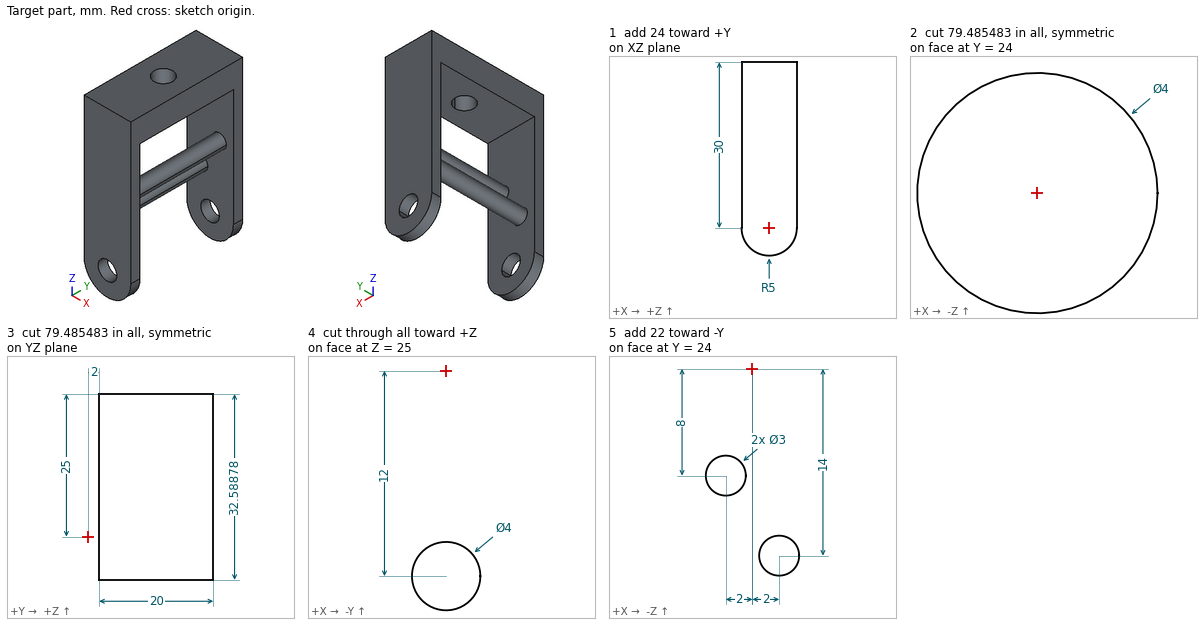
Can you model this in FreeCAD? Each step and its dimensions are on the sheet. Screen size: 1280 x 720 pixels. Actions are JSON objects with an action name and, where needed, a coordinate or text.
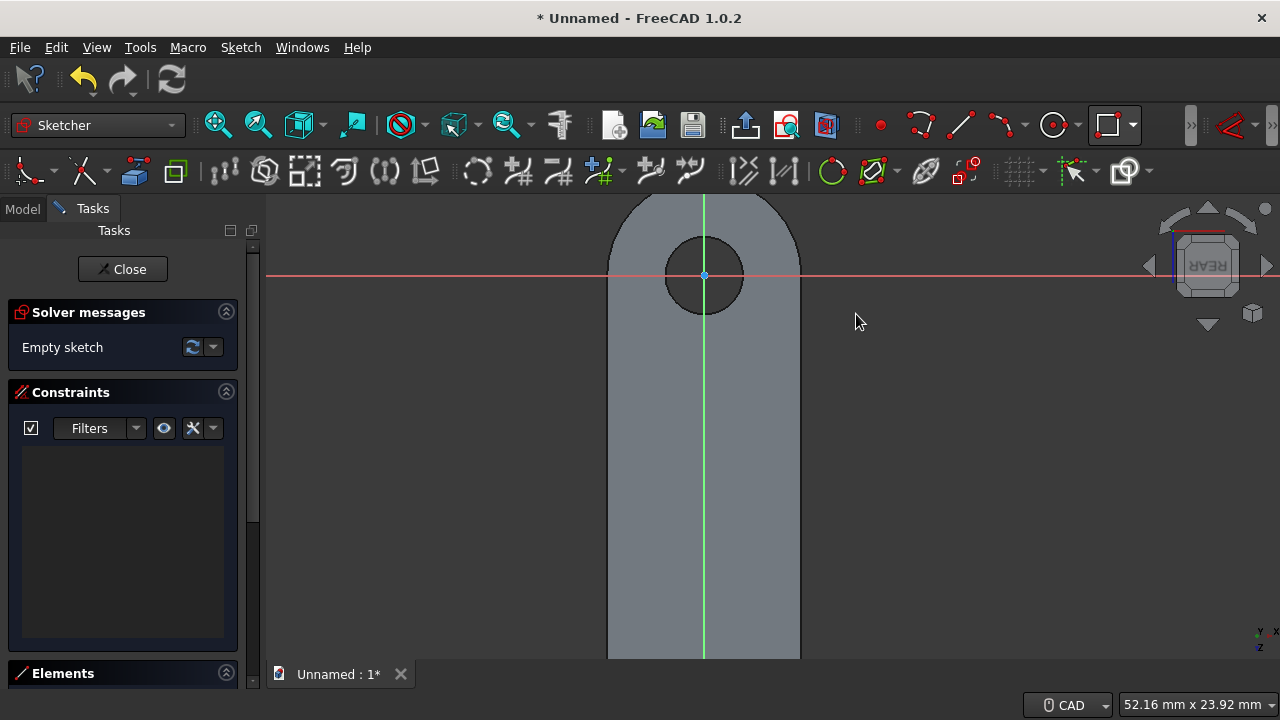
{"action": "left_click", "coordinate": [1054, 126]}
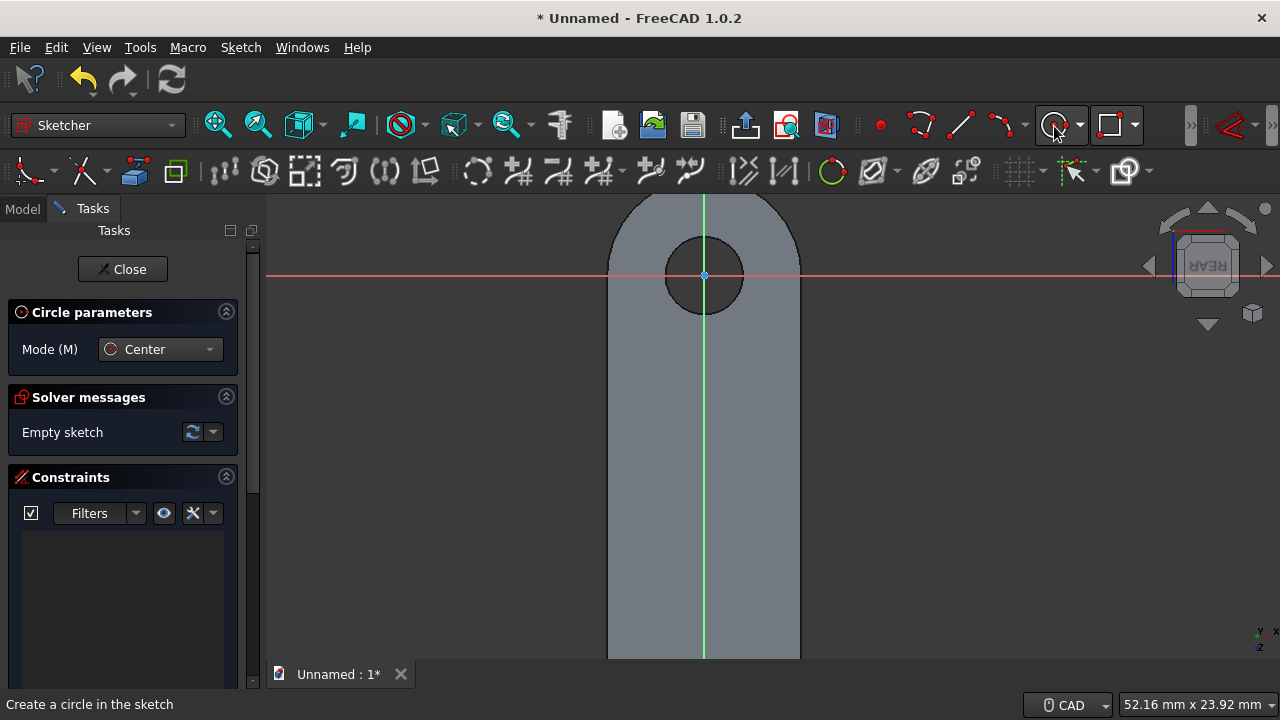
{"action": "left_click", "coordinate": [665, 431]}
{"action": "mouse_move", "coordinate": [686, 410]}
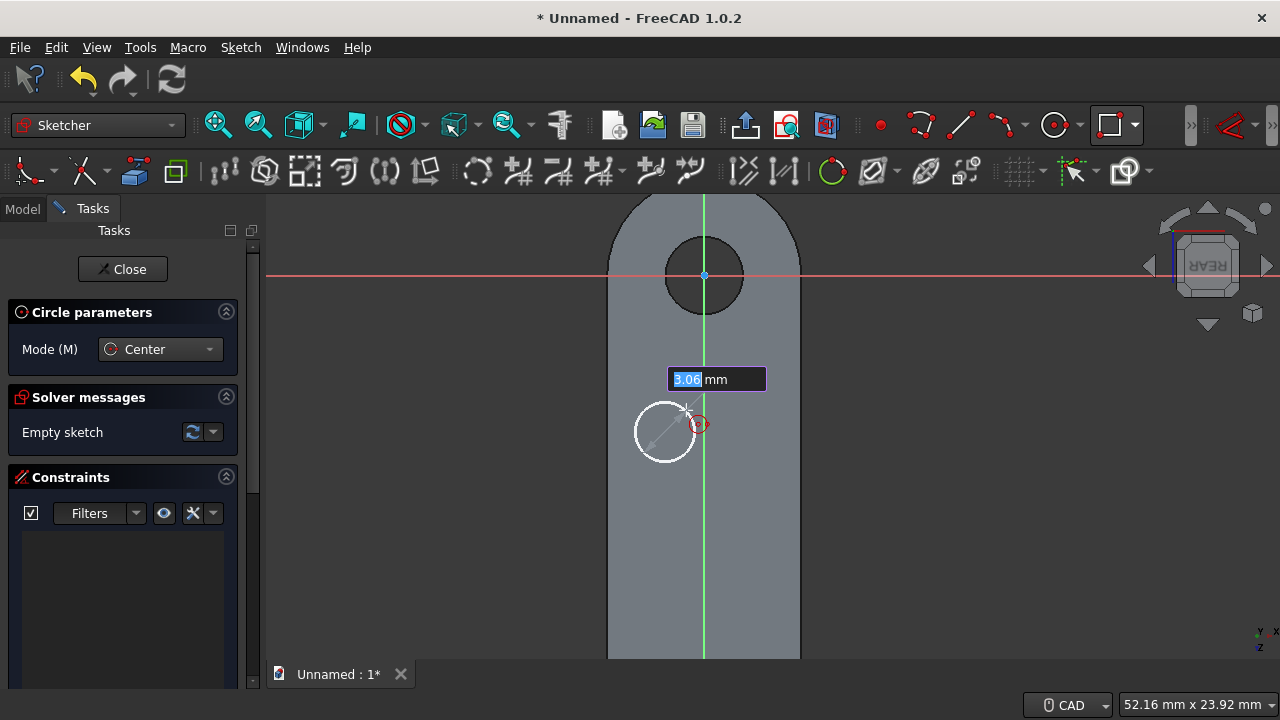
{"action": "type", "text": "3"}
{"action": "key", "text": "Return"}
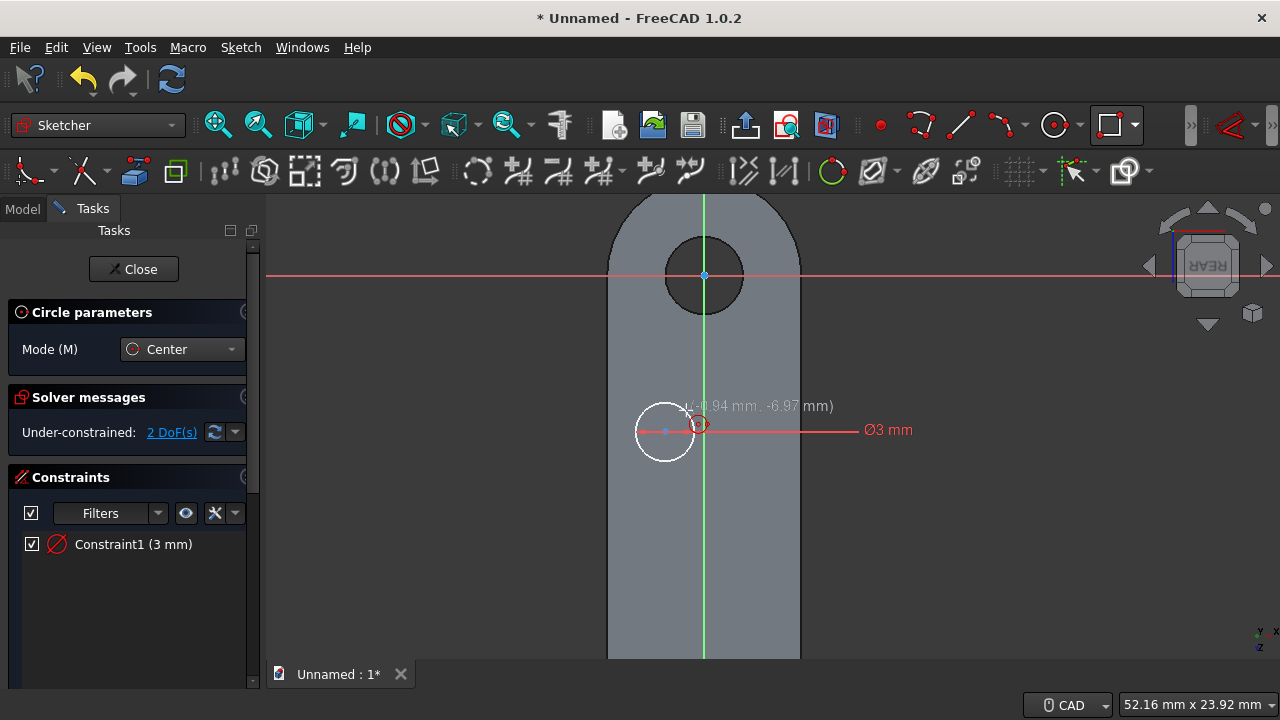
{"action": "left_click", "coordinate": [743, 548]}
{"action": "mouse_move", "coordinate": [764, 527]}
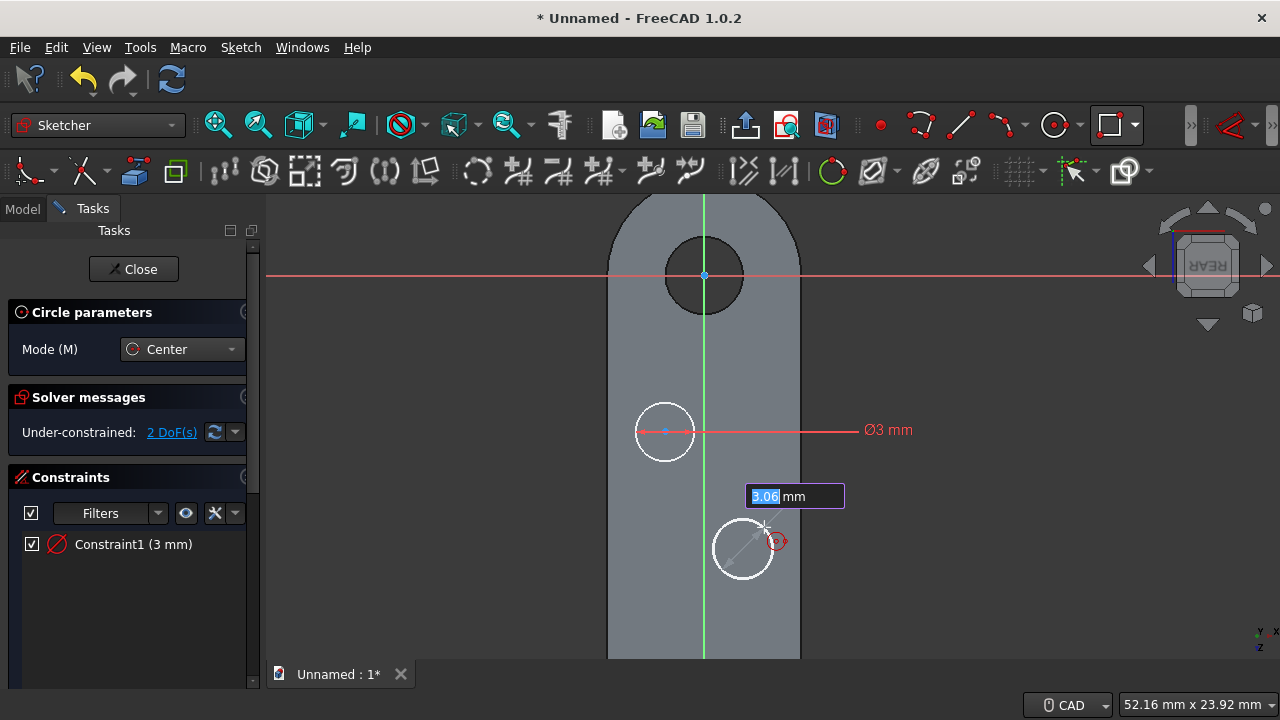
{"action": "type", "text": "3"}
{"action": "key", "text": "Return"}
{"action": "key", "text": "Escape"}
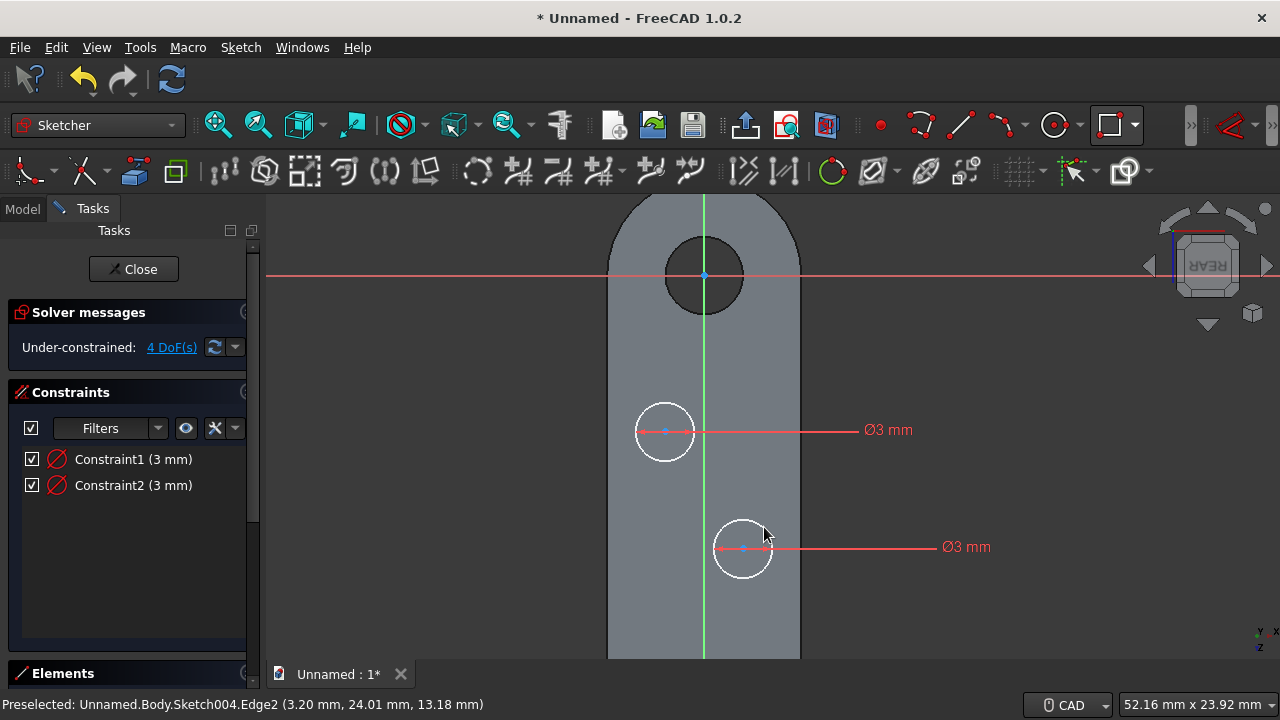
{"action": "left_click", "coordinate": [1230, 126]}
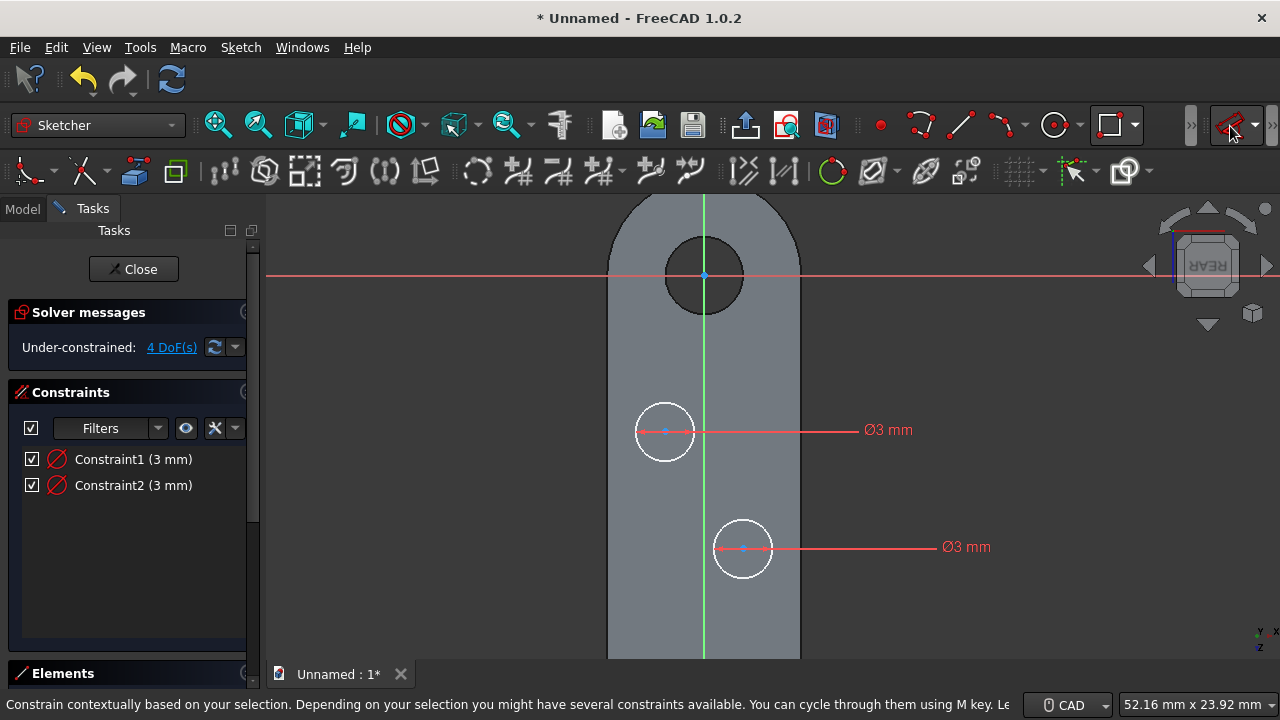
{"action": "left_click", "coordinate": [665, 432]}
{"action": "left_click", "coordinate": [685, 242]}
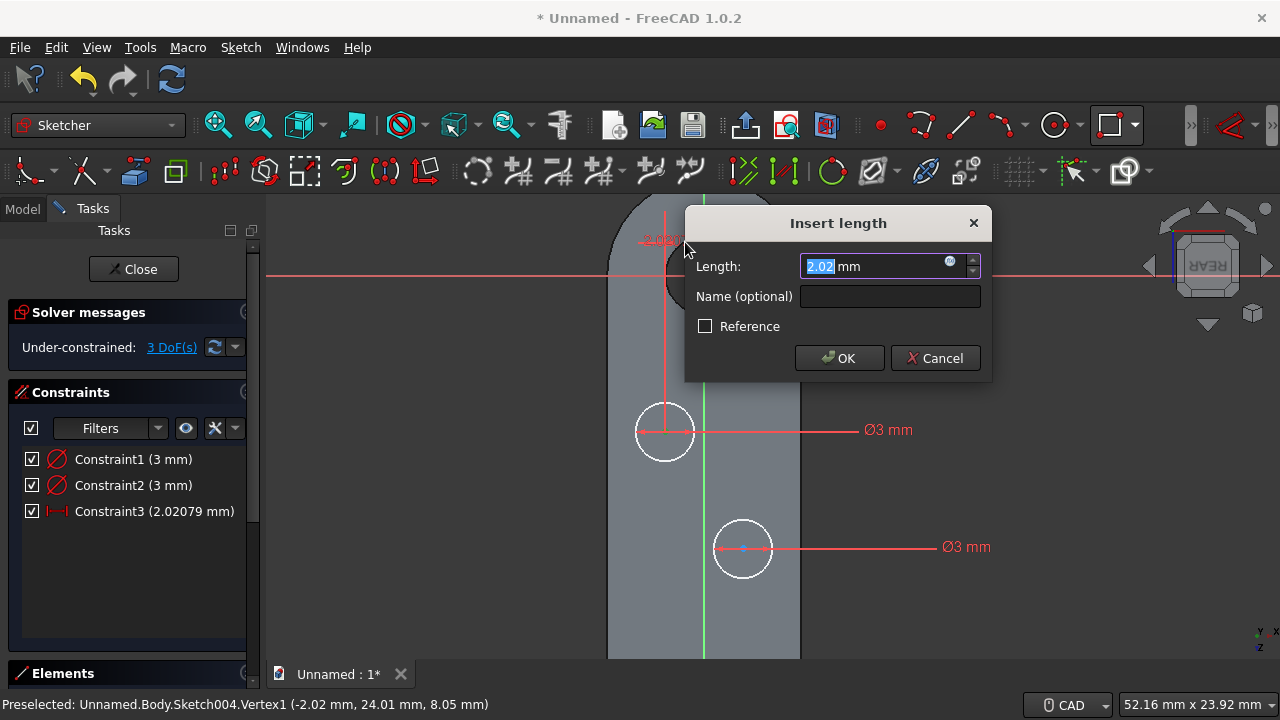
{"action": "type", "text": "2"}
{"action": "key", "text": "Return"}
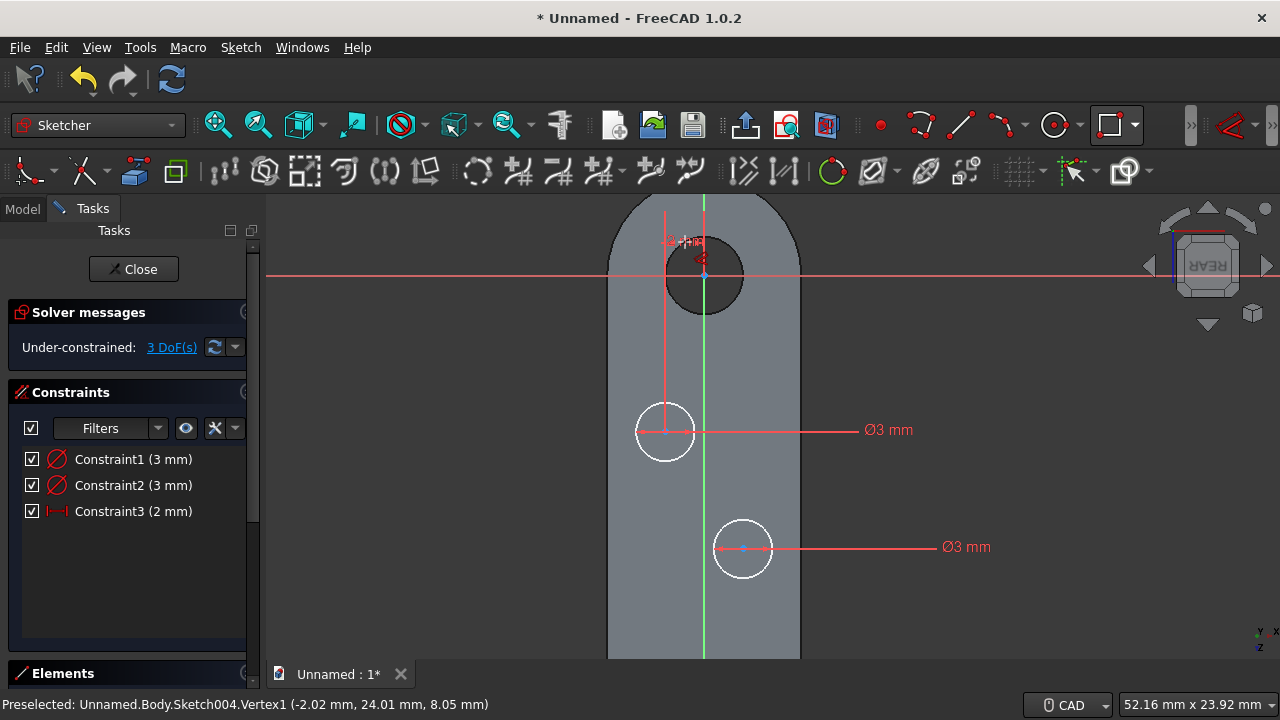
{"action": "left_click", "coordinate": [665, 432]}
{"action": "left_click", "coordinate": [631, 354]}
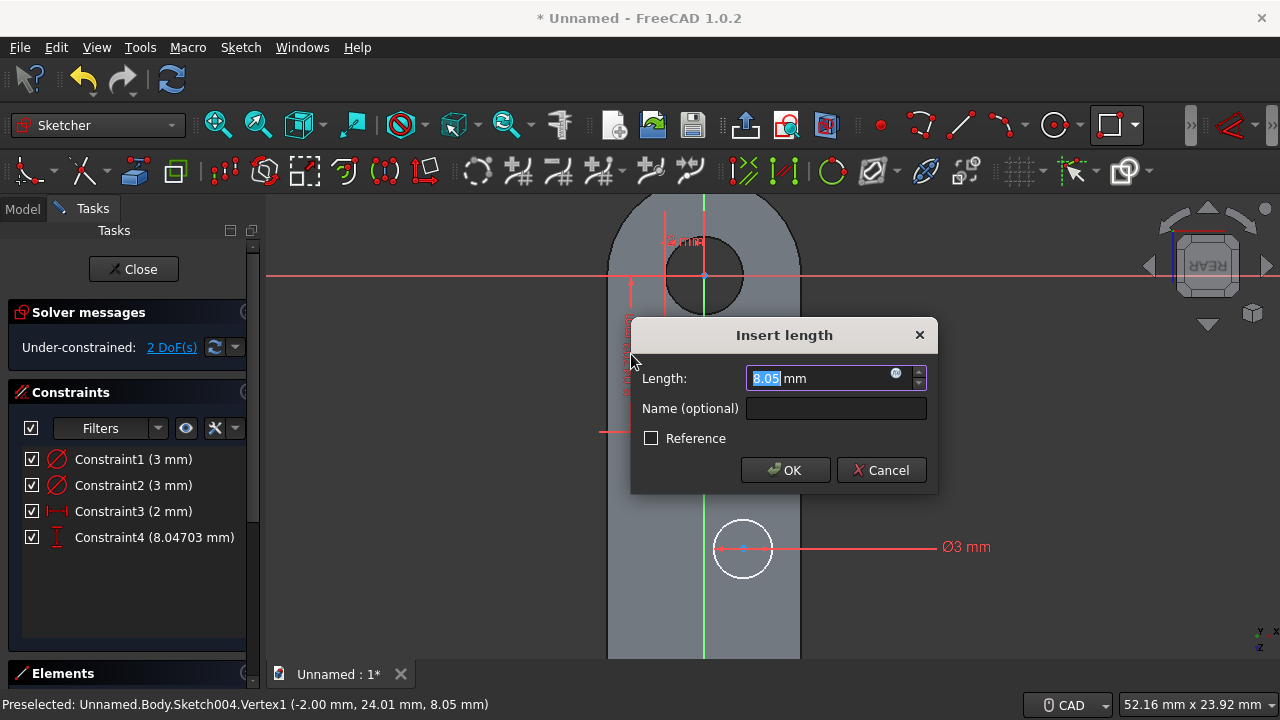
{"action": "type", "text": "8"}
{"action": "key", "text": "Return"}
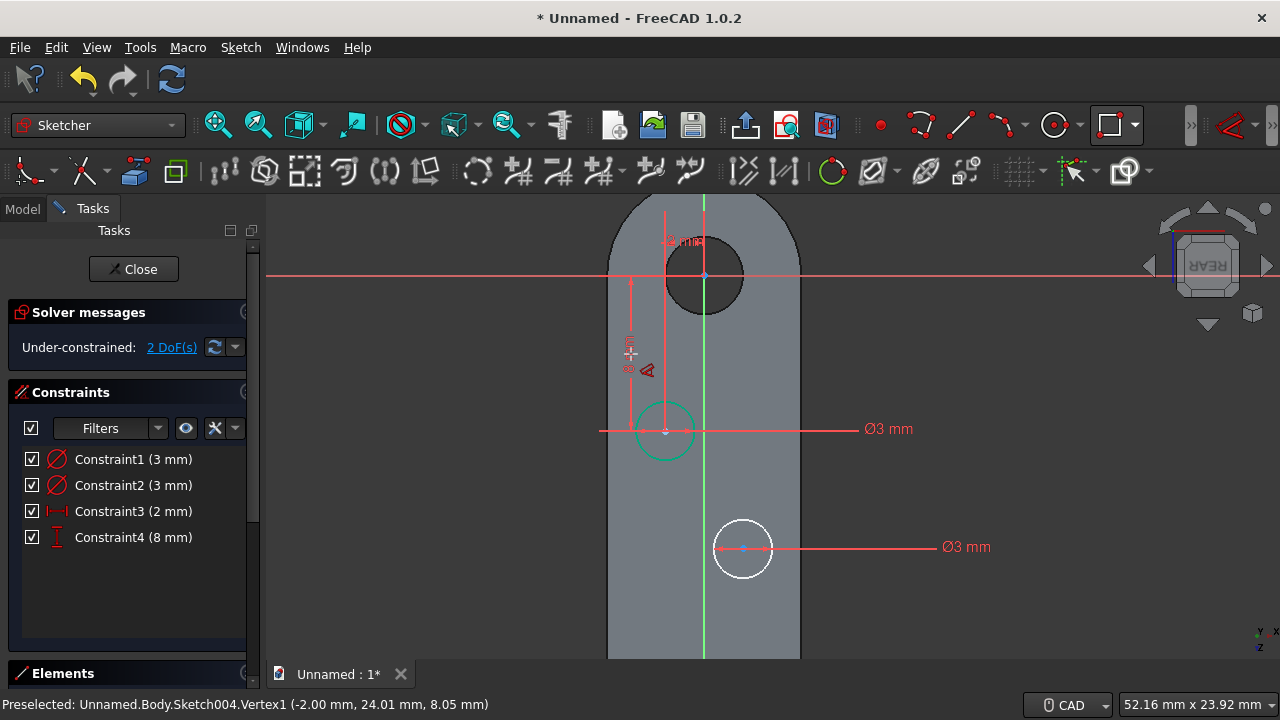
{"action": "left_click", "coordinate": [743, 549]}
{"action": "left_click", "coordinate": [724, 607]}